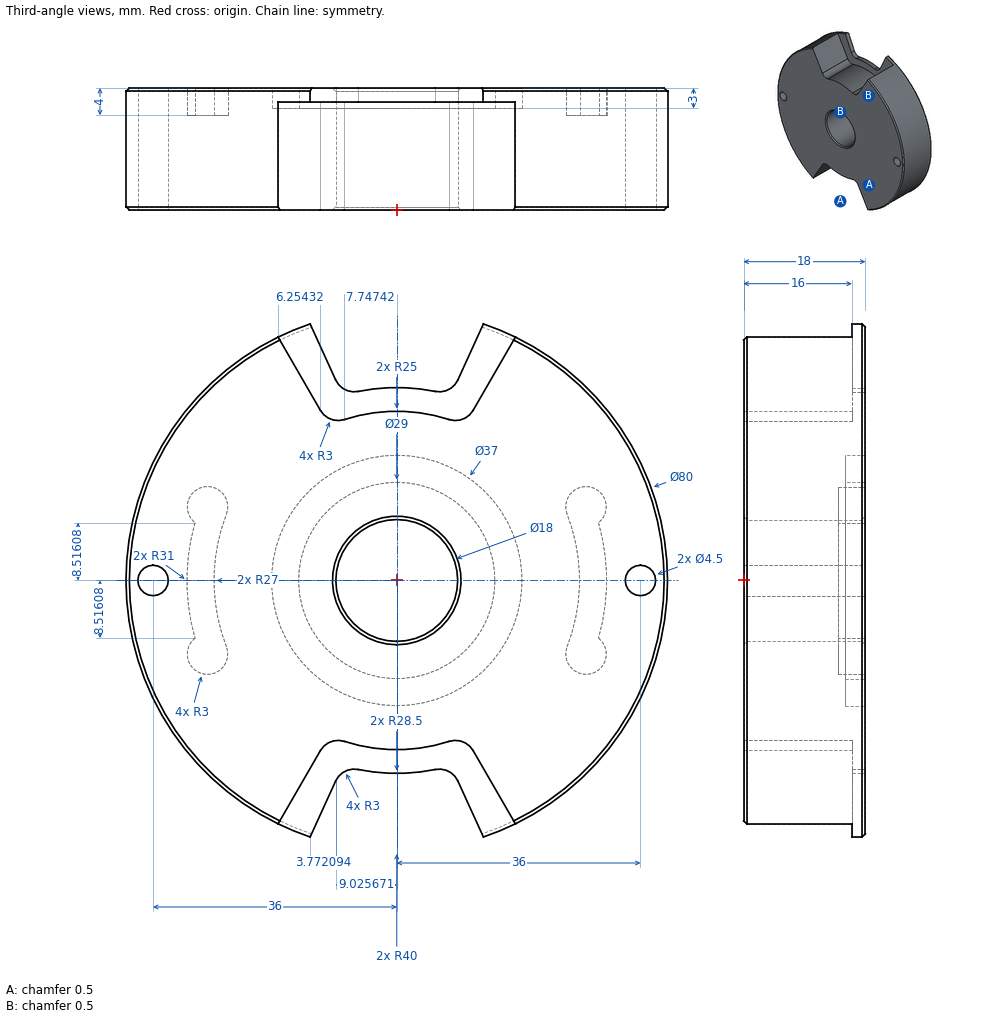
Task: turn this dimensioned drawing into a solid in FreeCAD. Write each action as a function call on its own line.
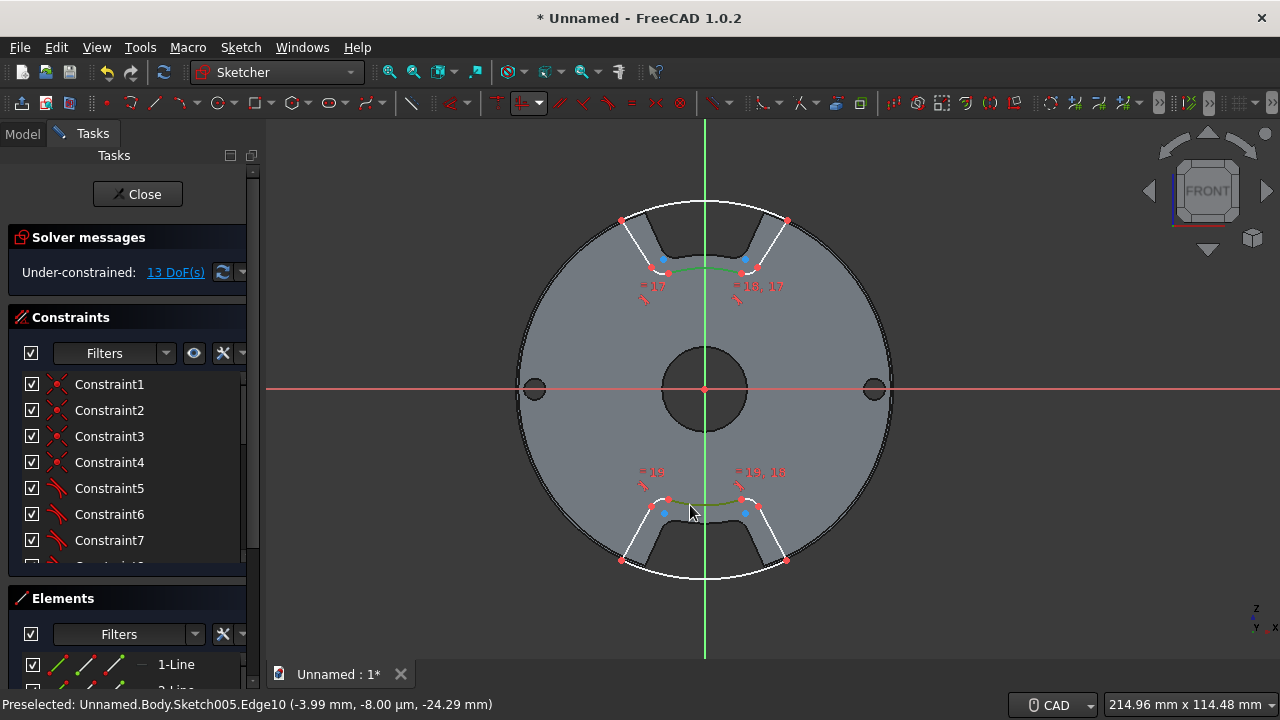
click(632, 104)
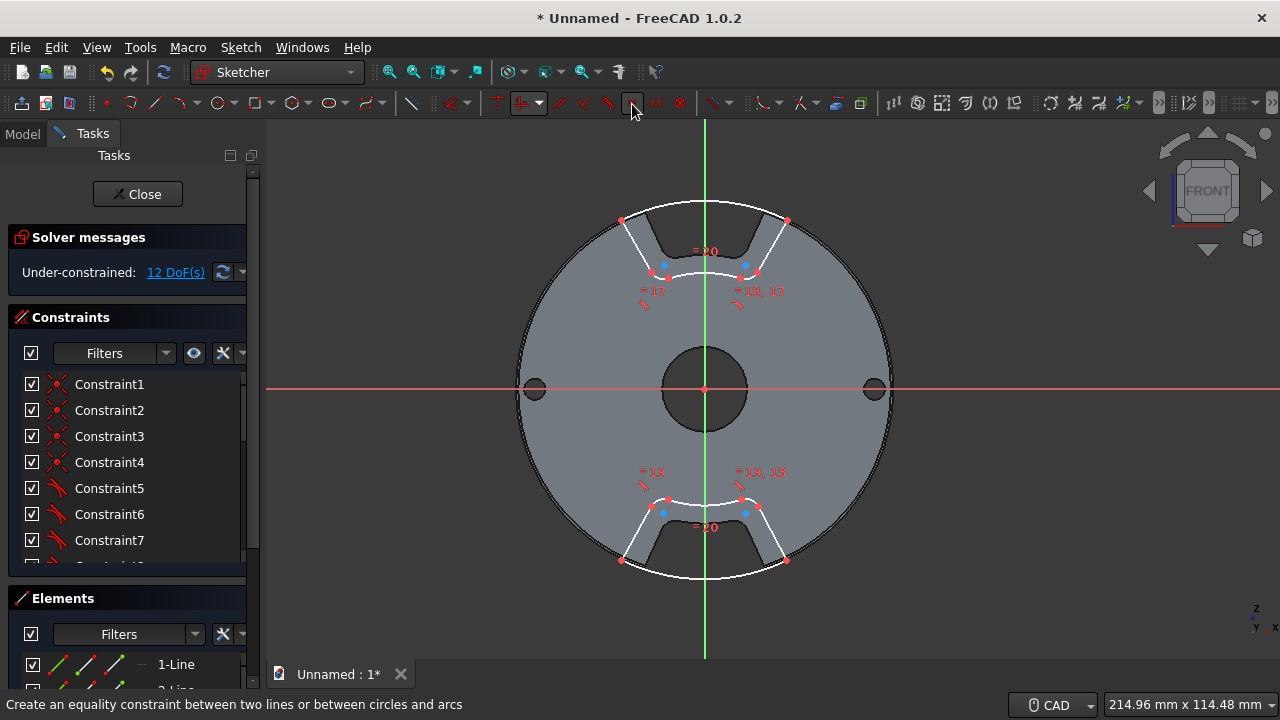
click(739, 204)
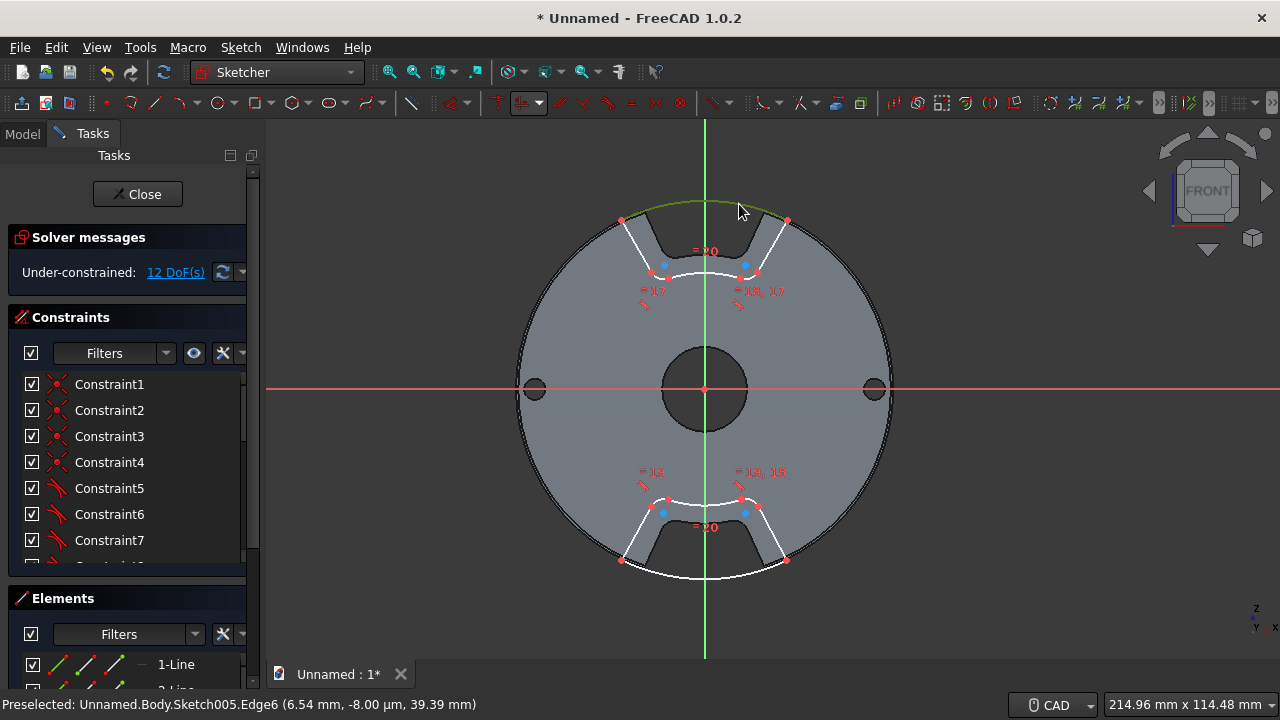
click(670, 576)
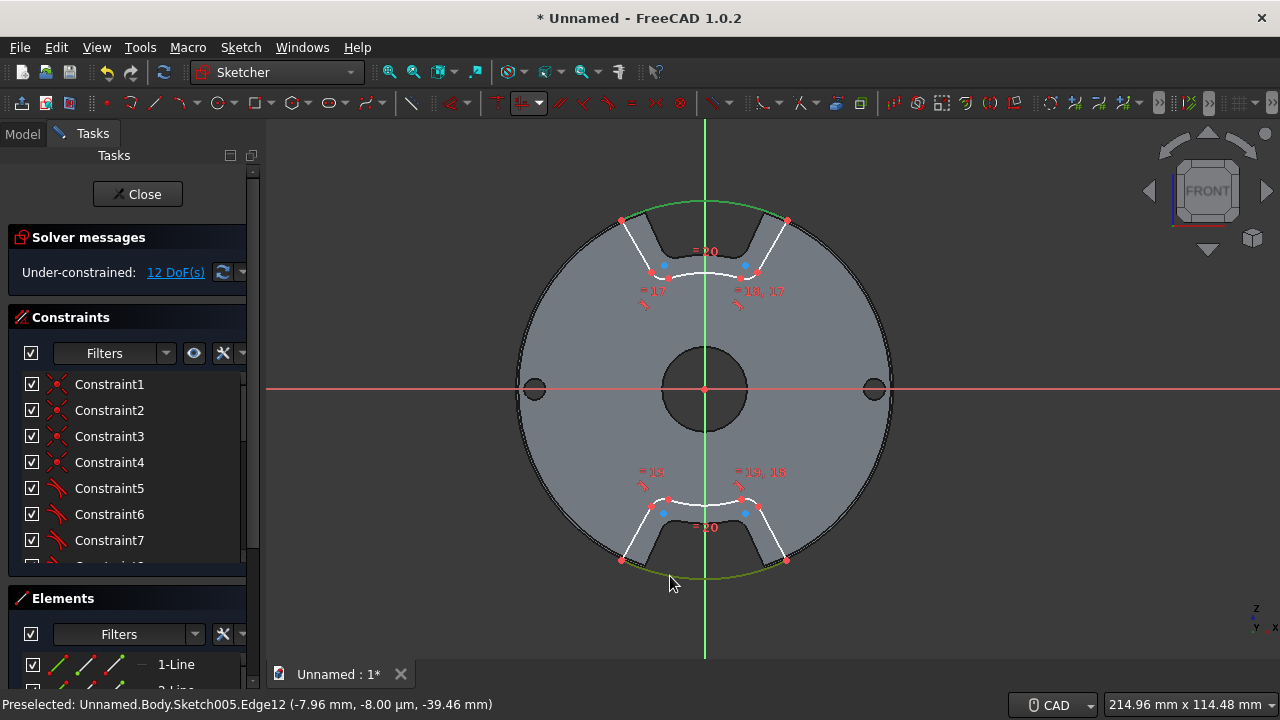
click(632, 104)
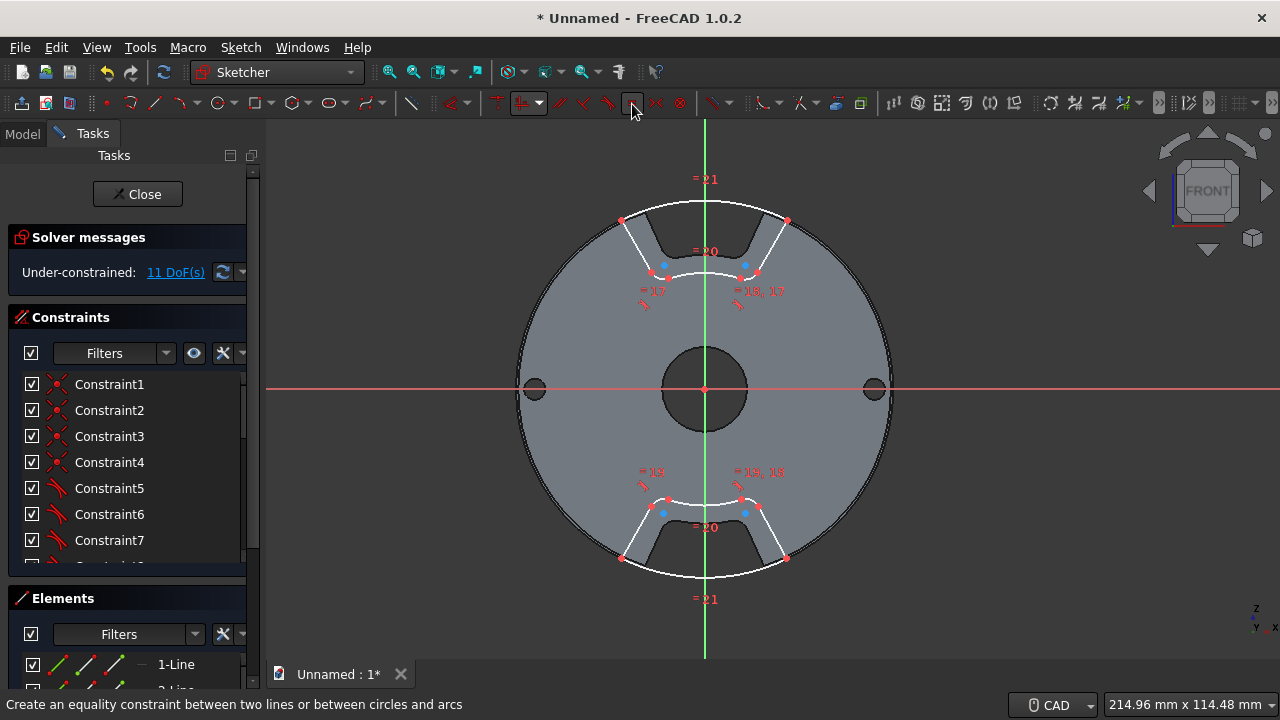
click(652, 272)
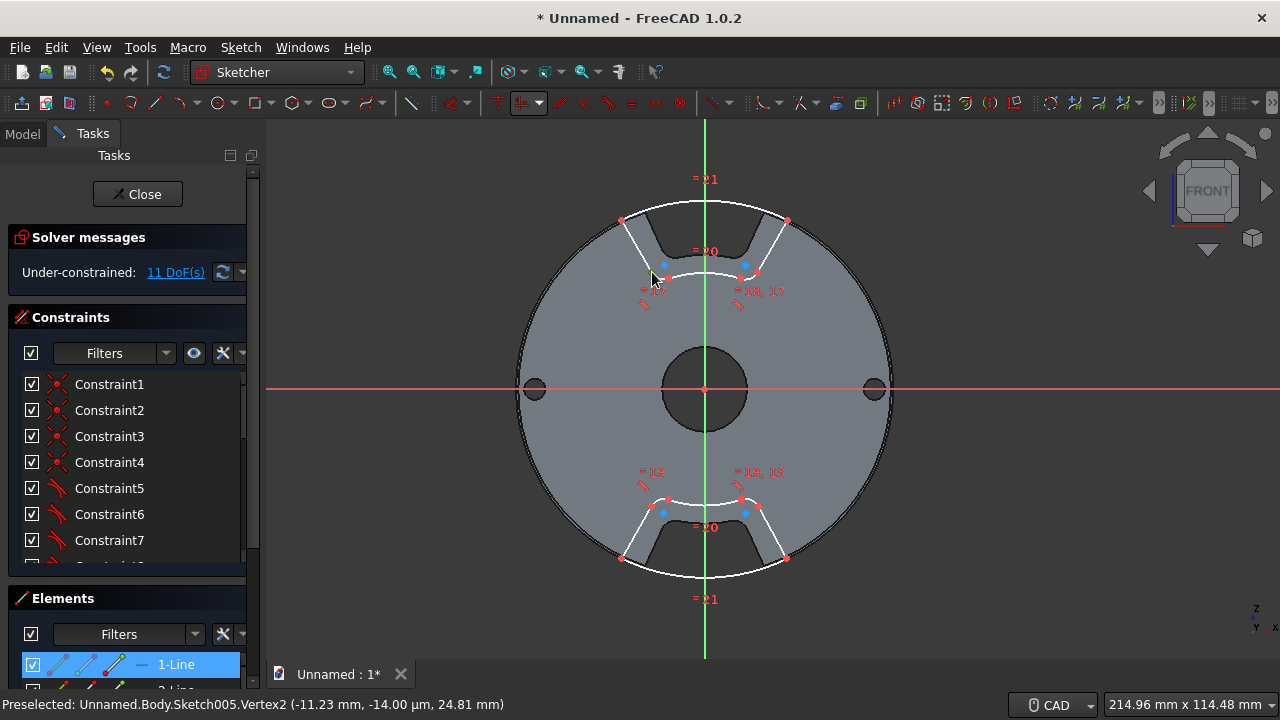
click(758, 272)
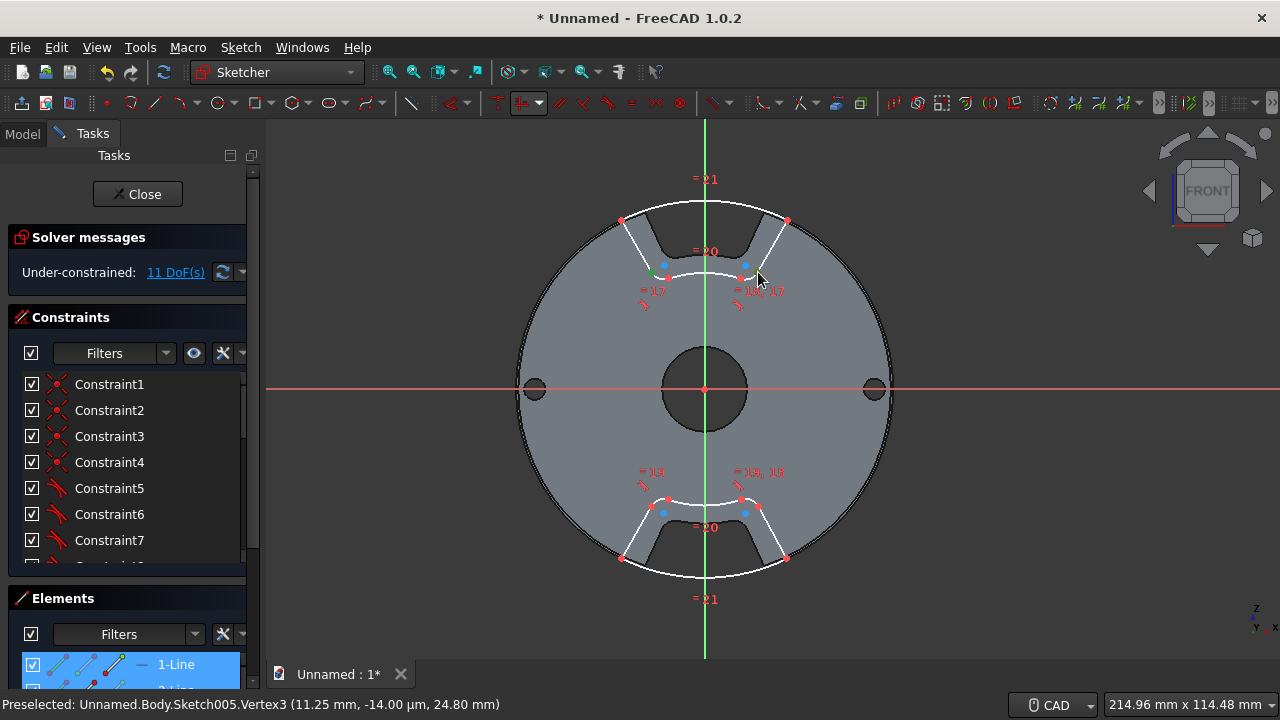
click(705, 458)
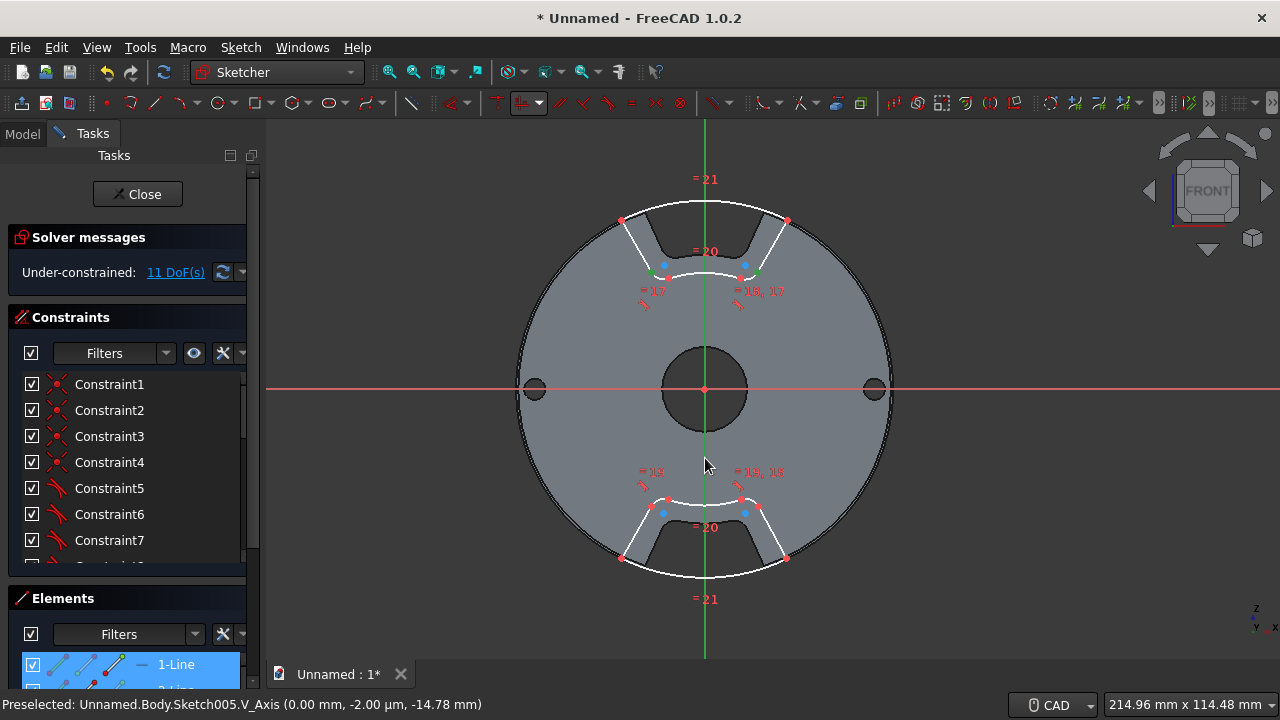
click(656, 104)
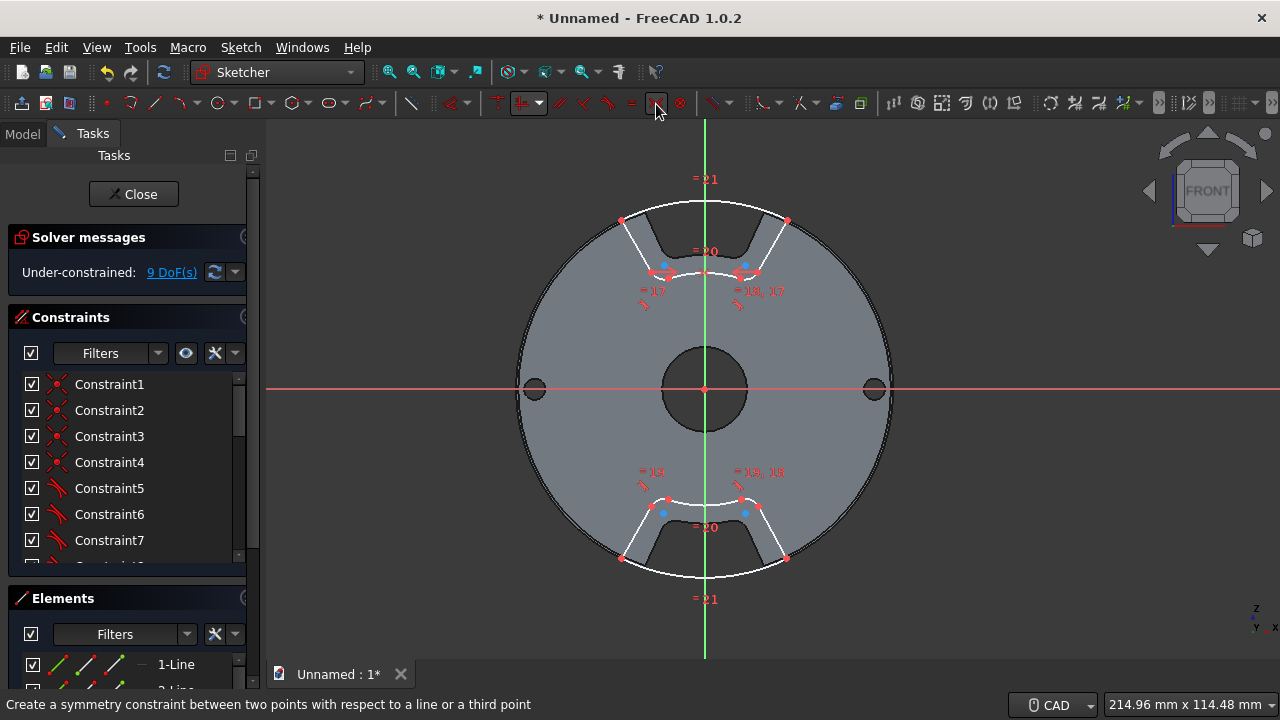
click(758, 272)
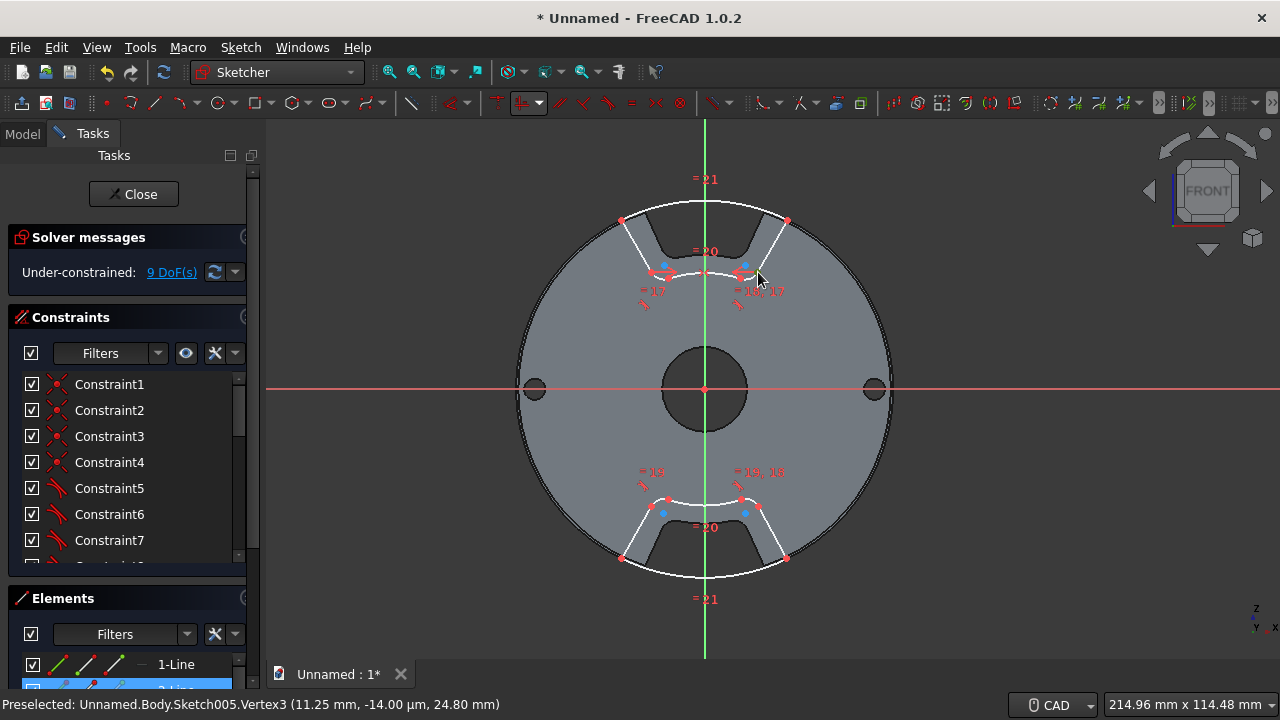
click(758, 506)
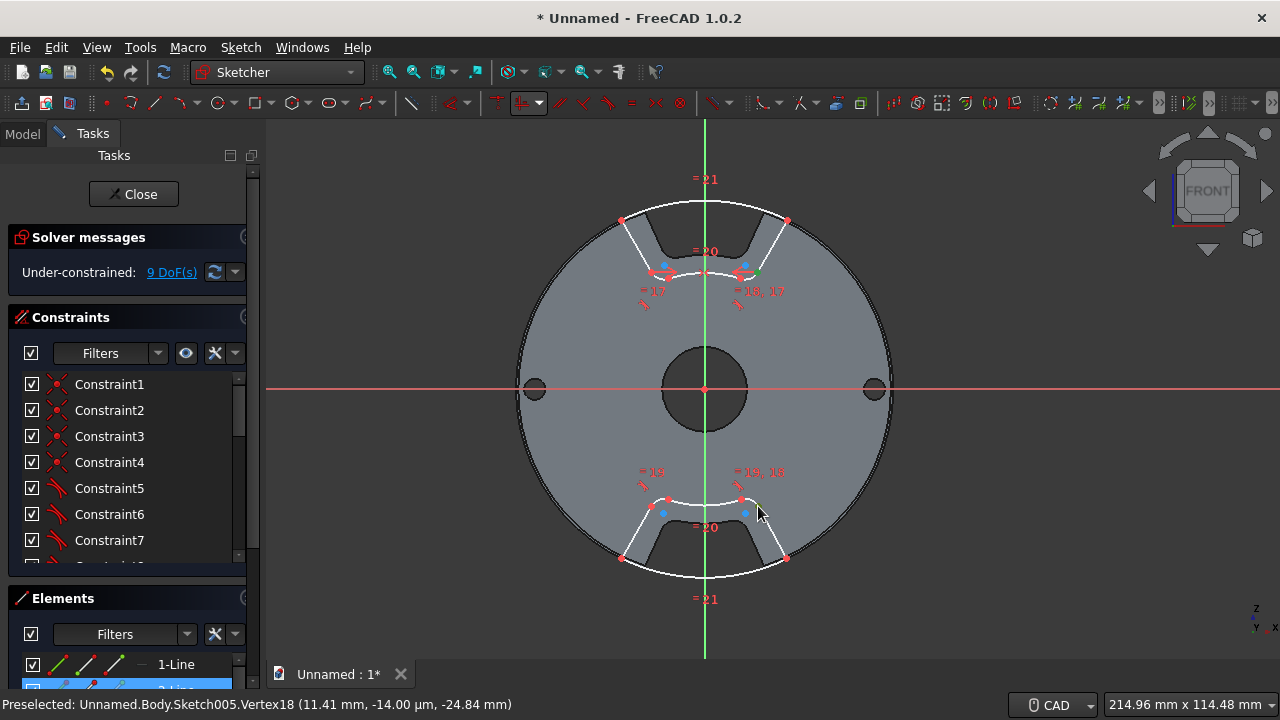
click(353, 389)